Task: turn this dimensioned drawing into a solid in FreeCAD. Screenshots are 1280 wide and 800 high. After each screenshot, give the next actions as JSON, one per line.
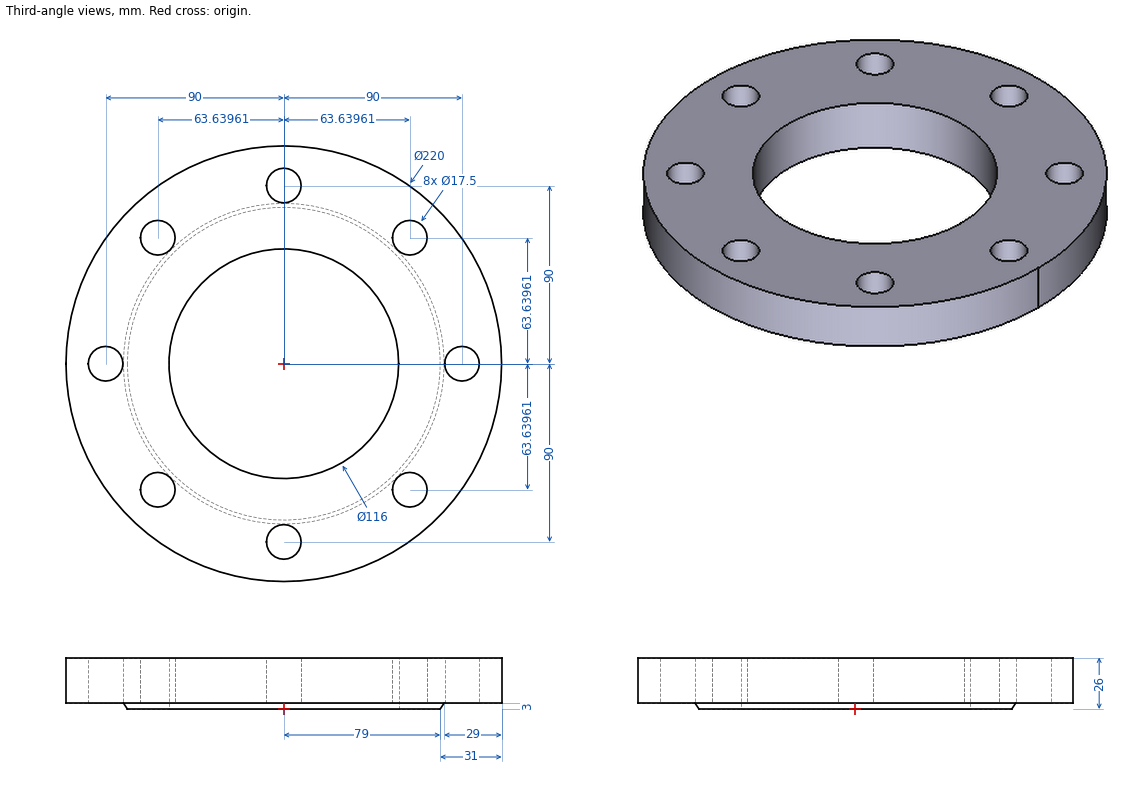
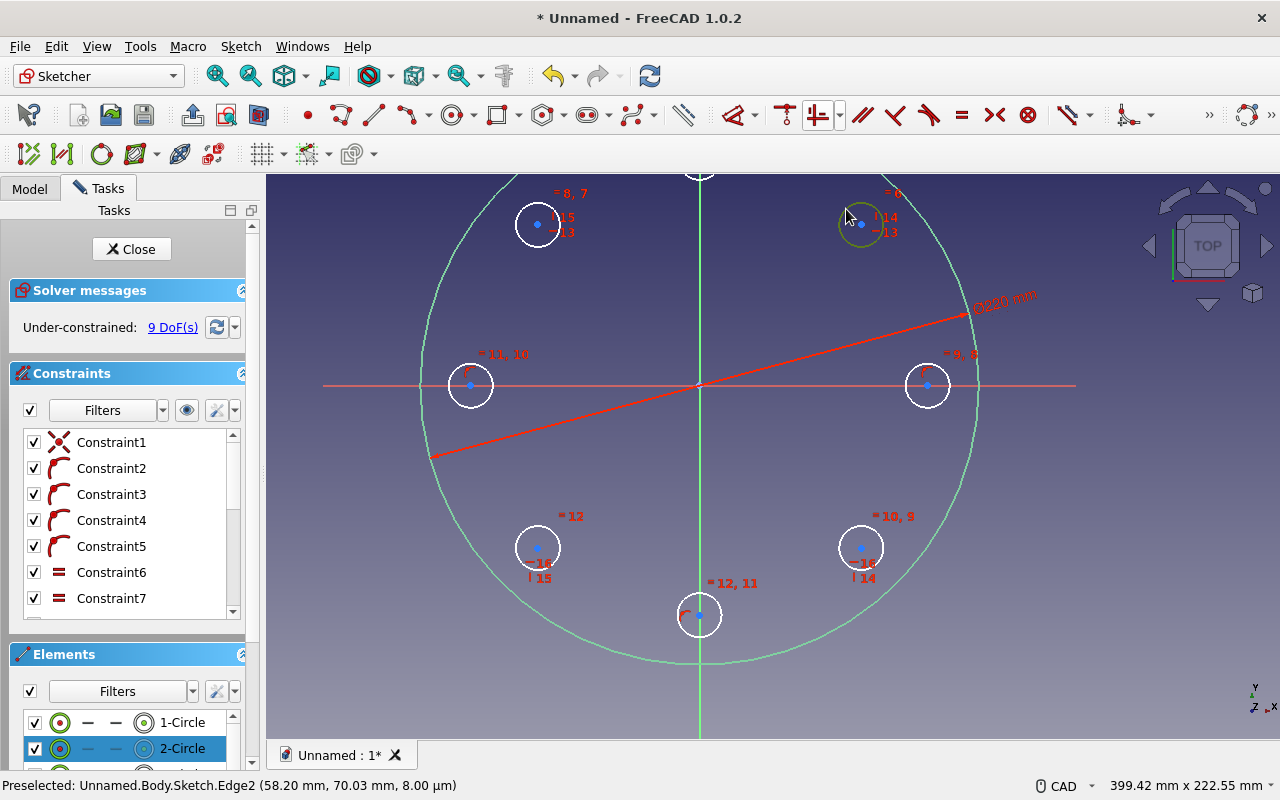
{"action": "key", "text": "k o"}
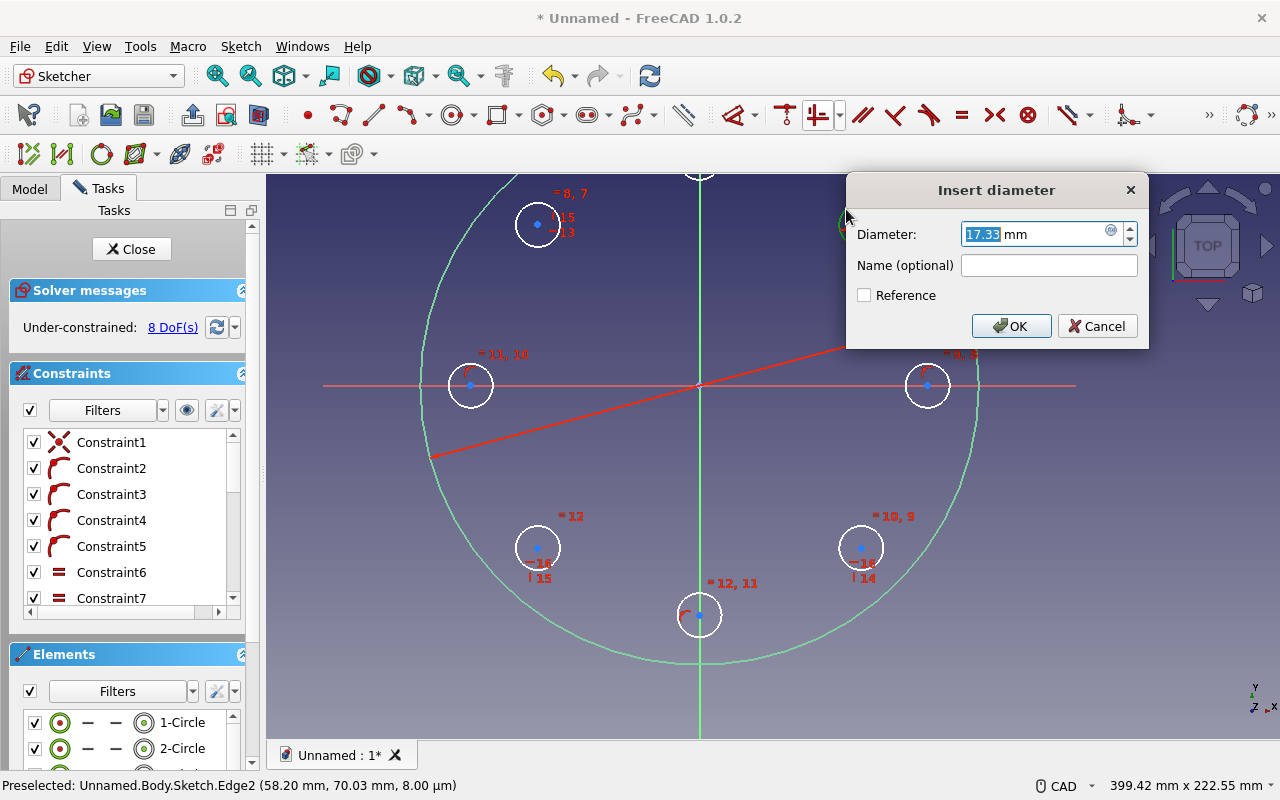
{"action": "type", "text": "17.5"}
{"action": "key", "text": "Return"}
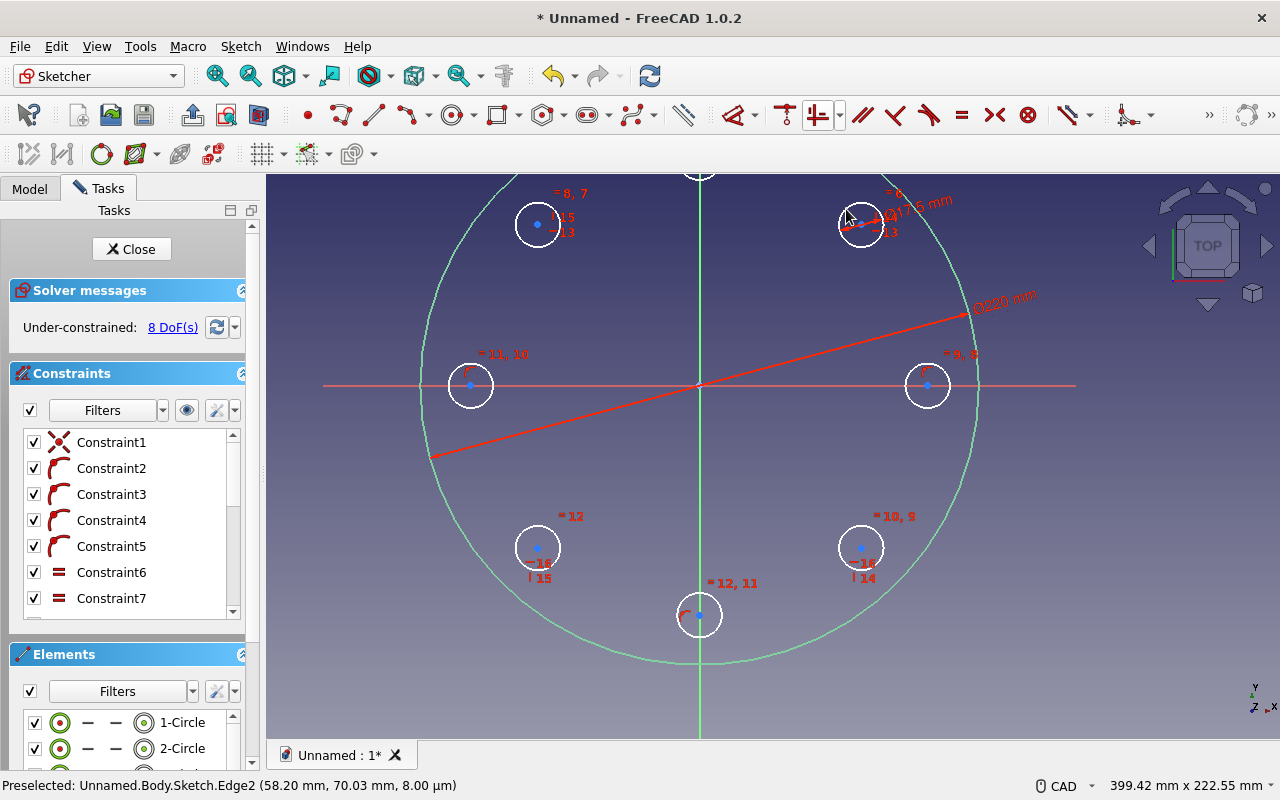
{"action": "scroll", "coordinate": [715, 600], "scroll_direction": "down", "scroll_amount": 2}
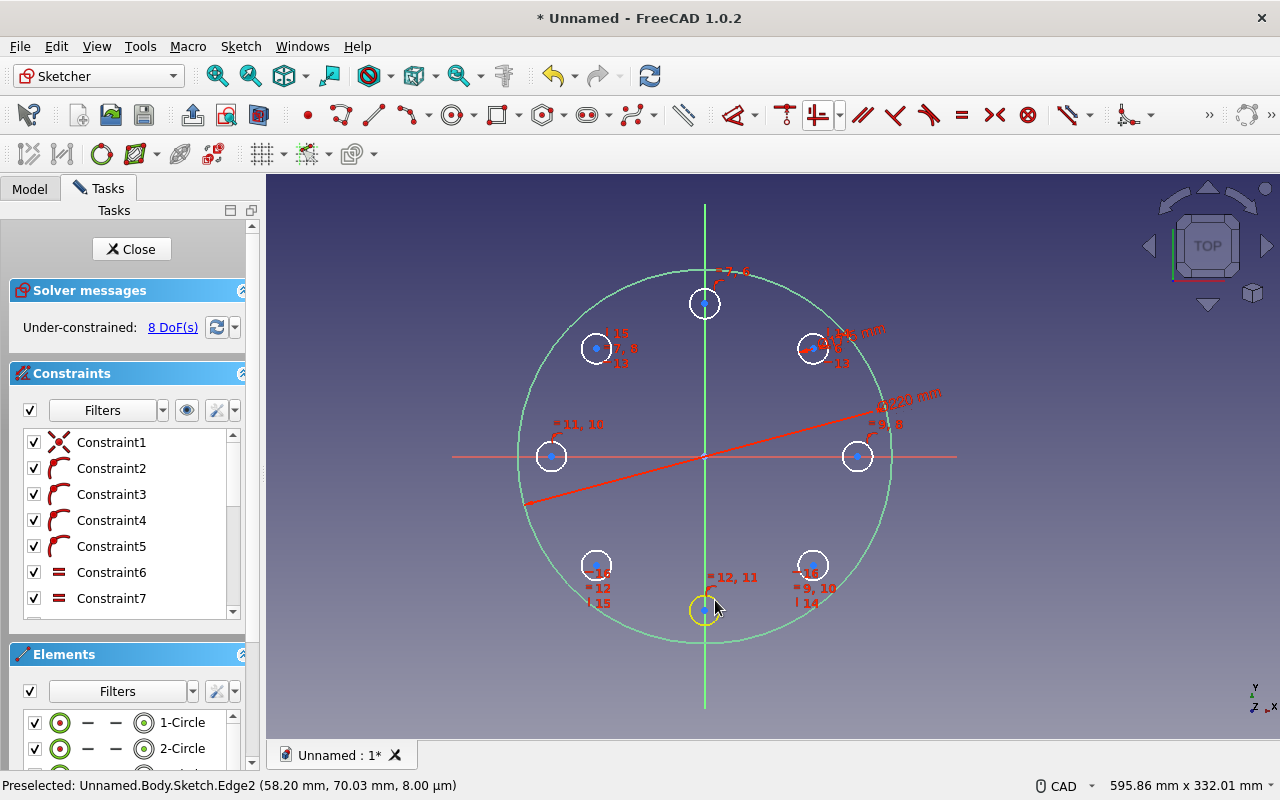
{"action": "left_click", "coordinate": [705, 304]}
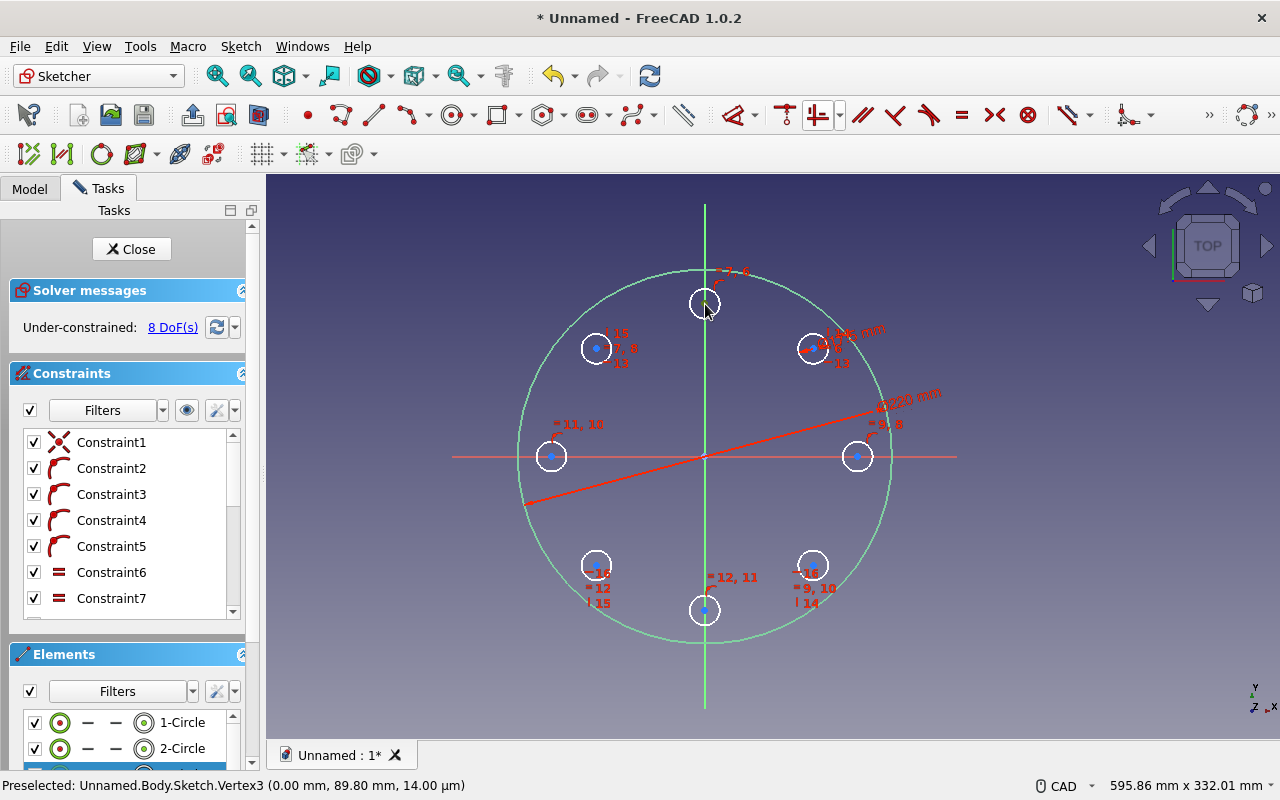
{"action": "key", "text": "i"}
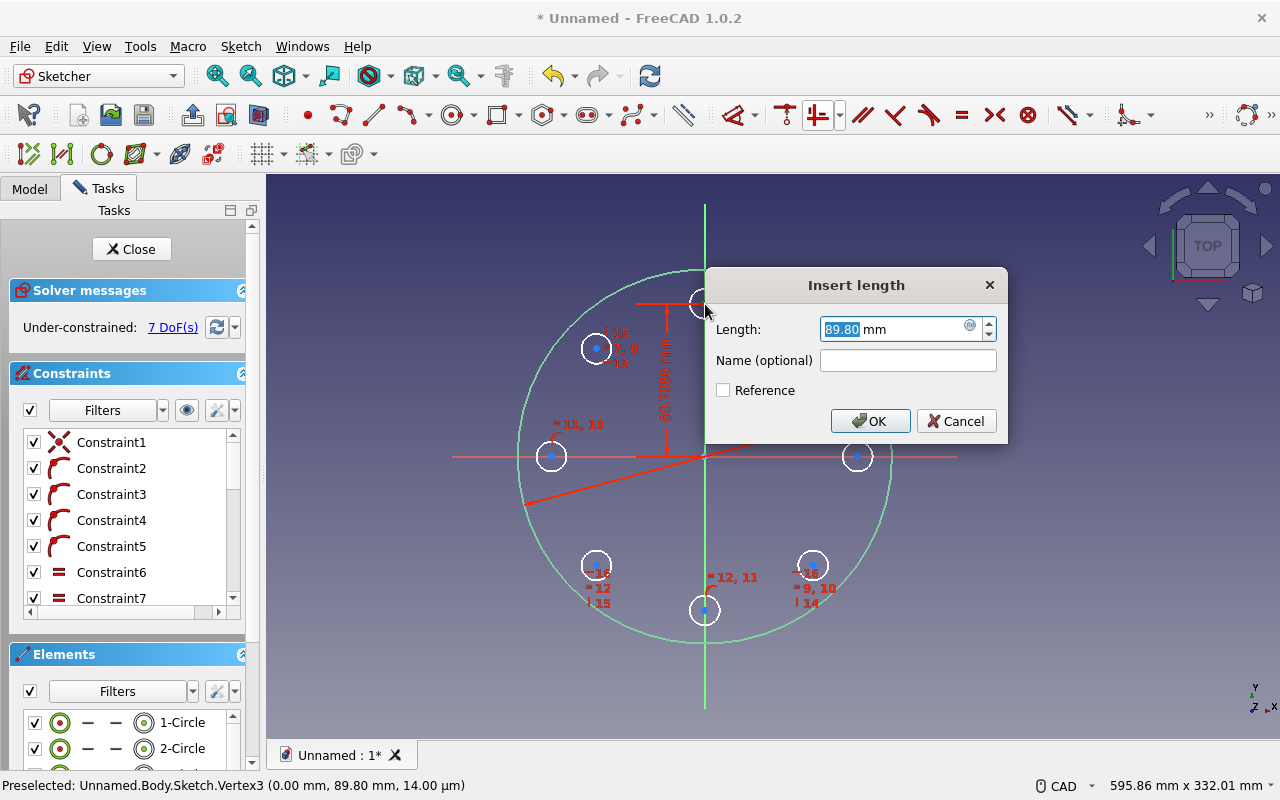
{"action": "type", "text": "90"}
{"action": "key", "text": "Return"}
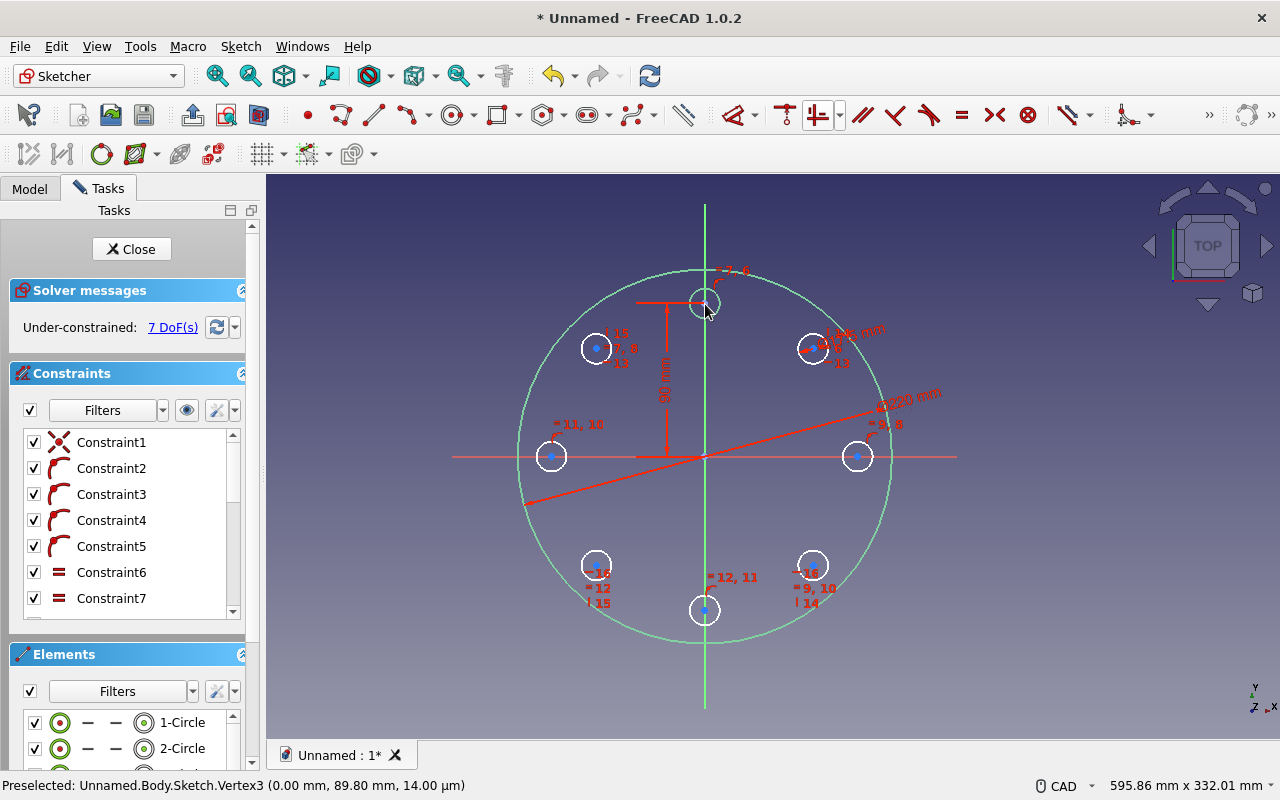
{"action": "left_click", "coordinate": [858, 457]}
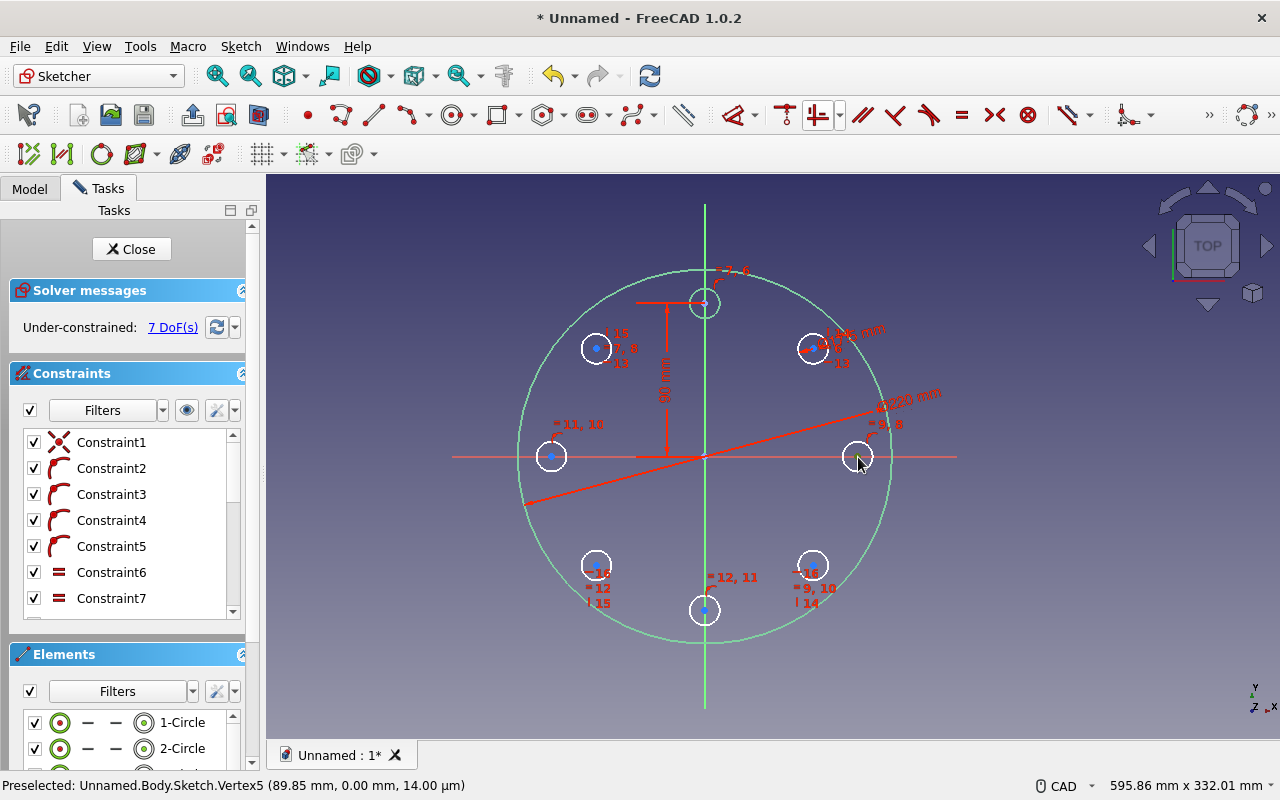
{"action": "left_click", "coordinate": [754, 116]}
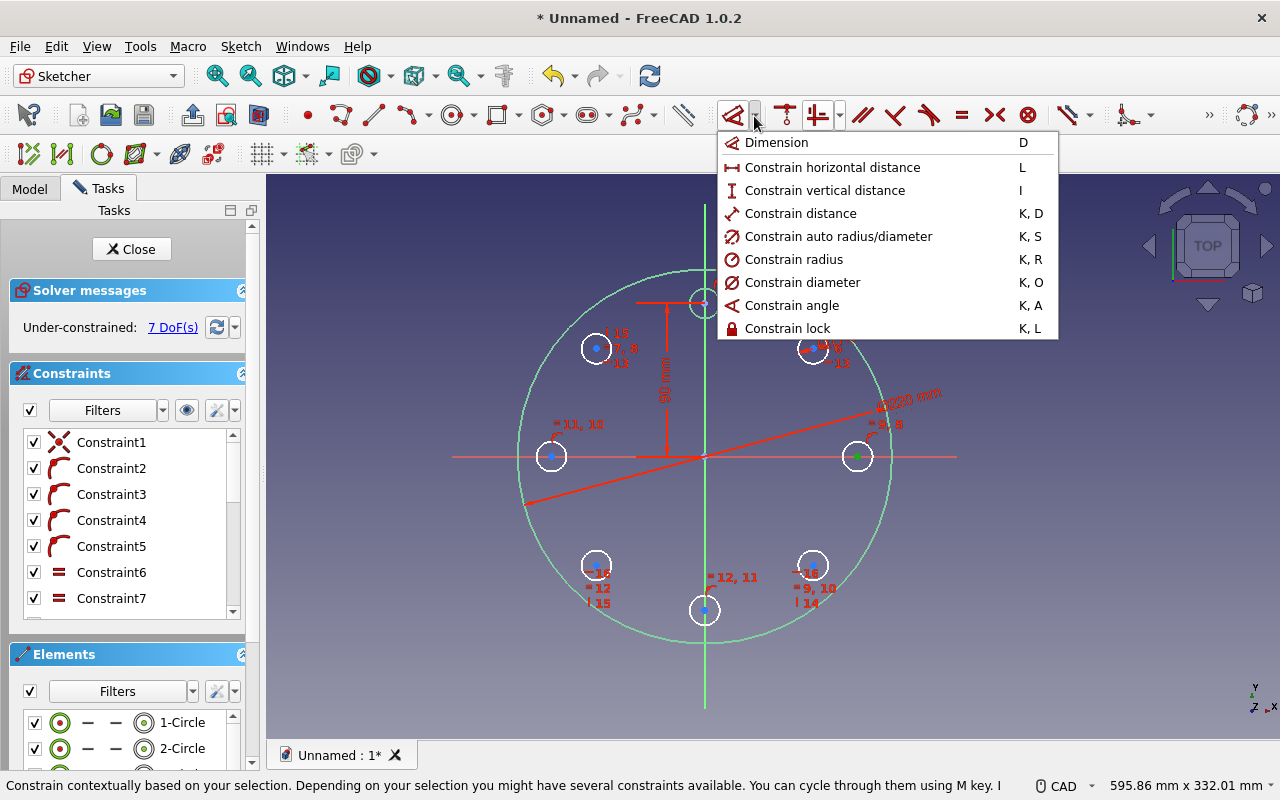
{"action": "left_click", "coordinate": [888, 168]}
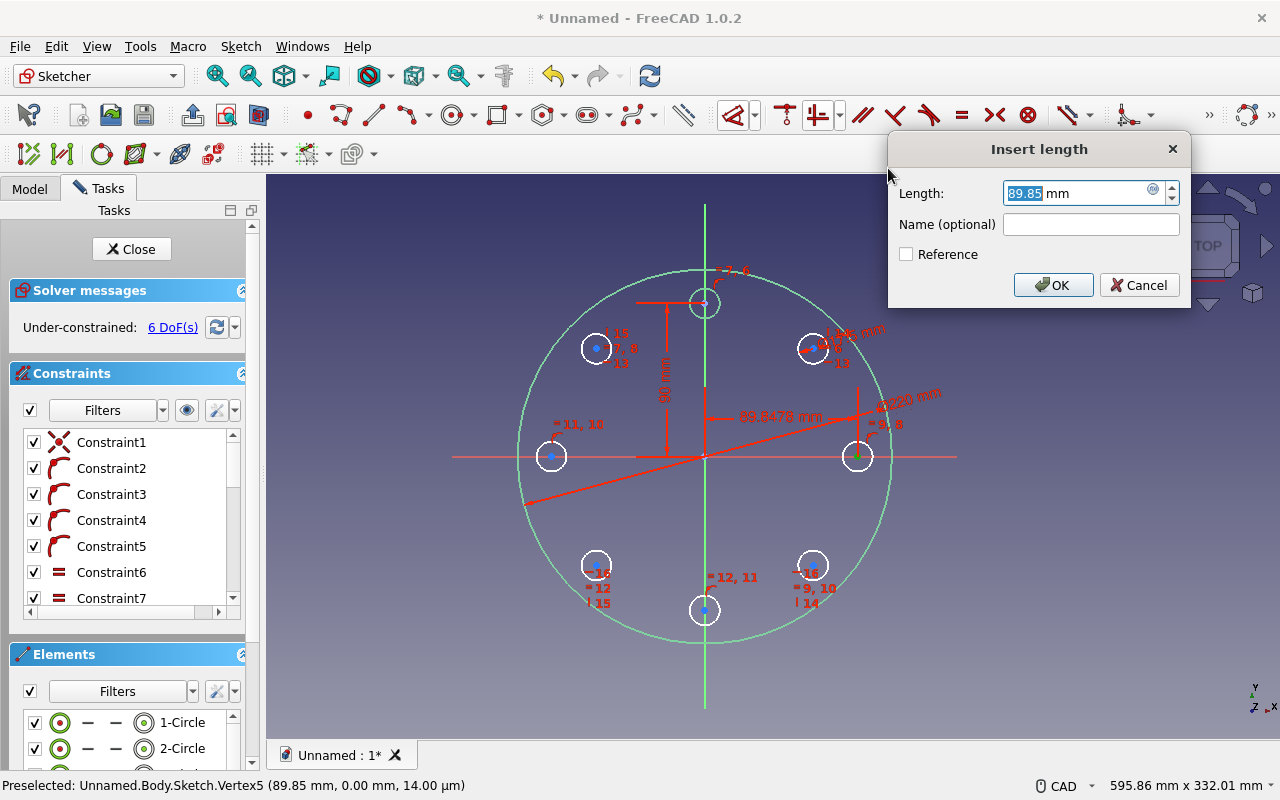
{"action": "type", "text": "90"}
{"action": "key", "text": "Return"}